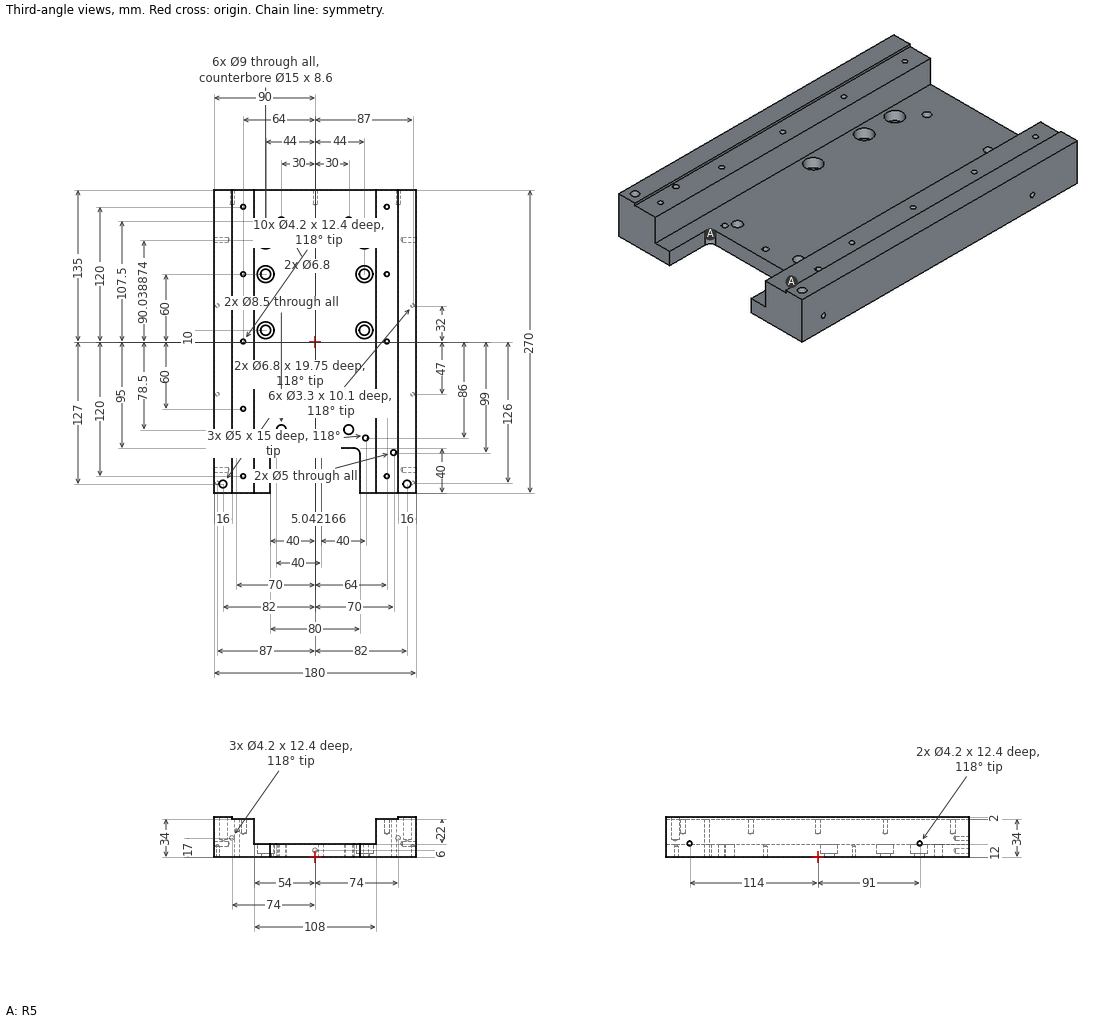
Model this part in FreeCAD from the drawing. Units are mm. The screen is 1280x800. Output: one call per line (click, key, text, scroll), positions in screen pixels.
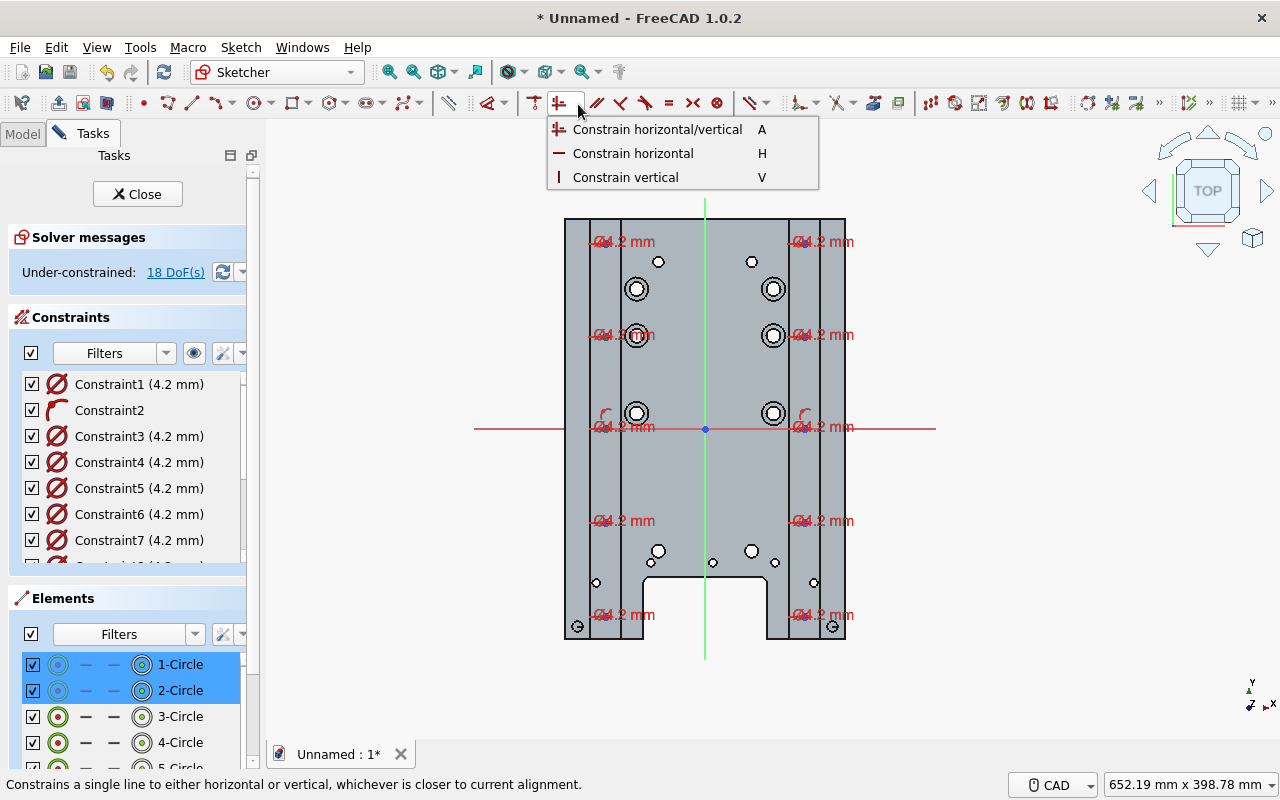
click(683, 177)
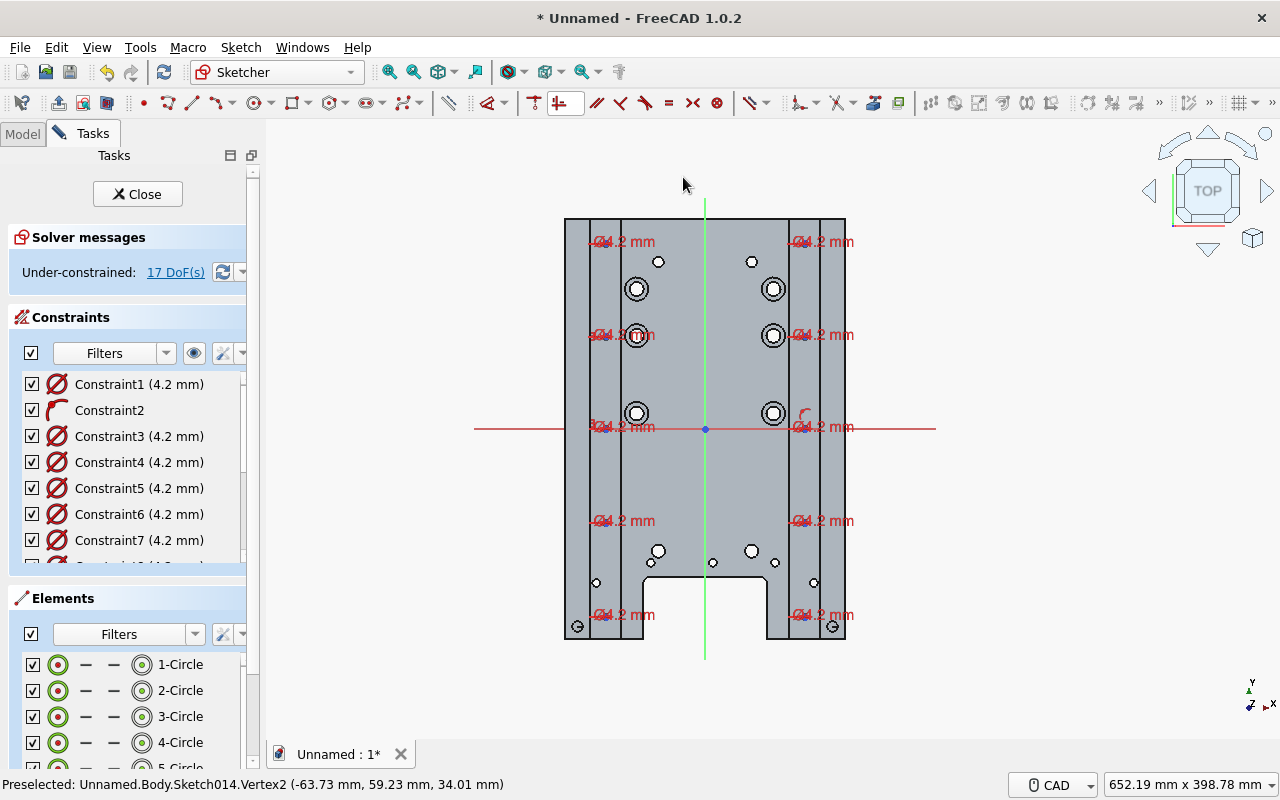
click(606, 337)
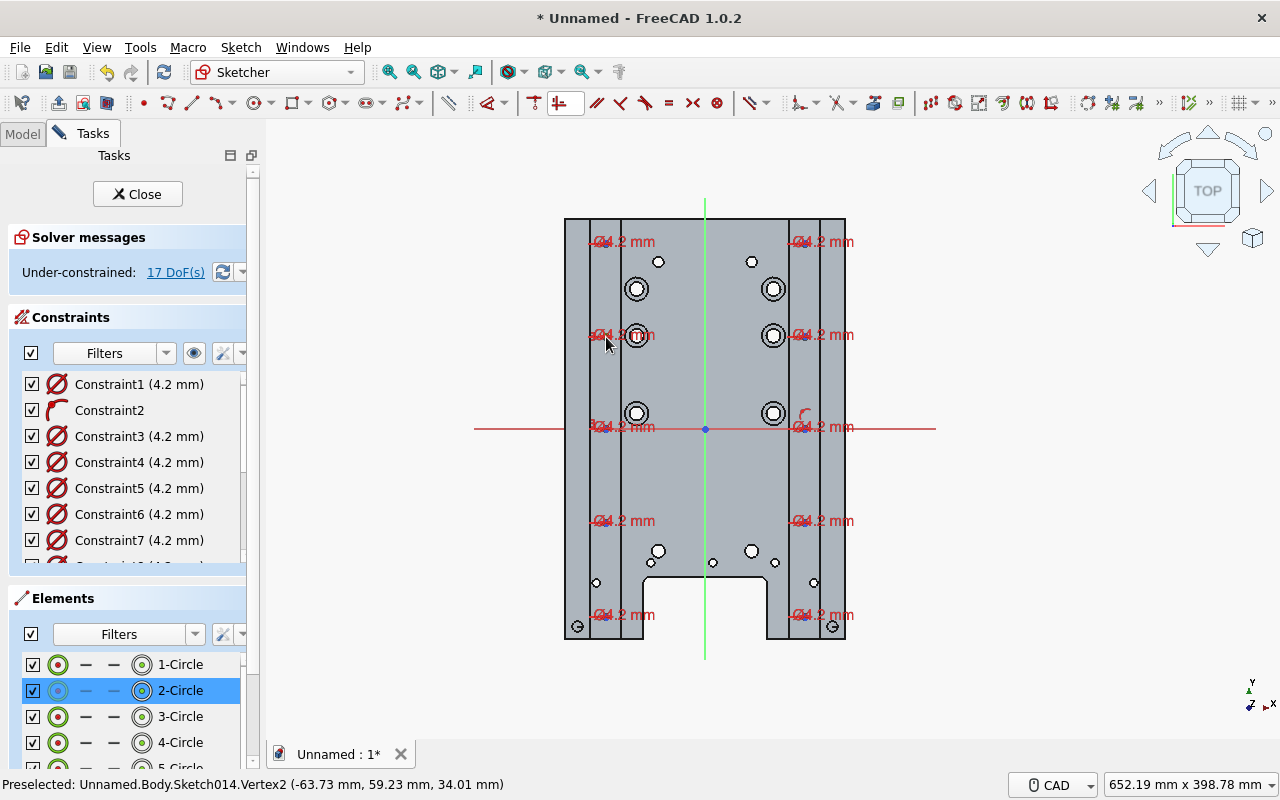
click(606, 244)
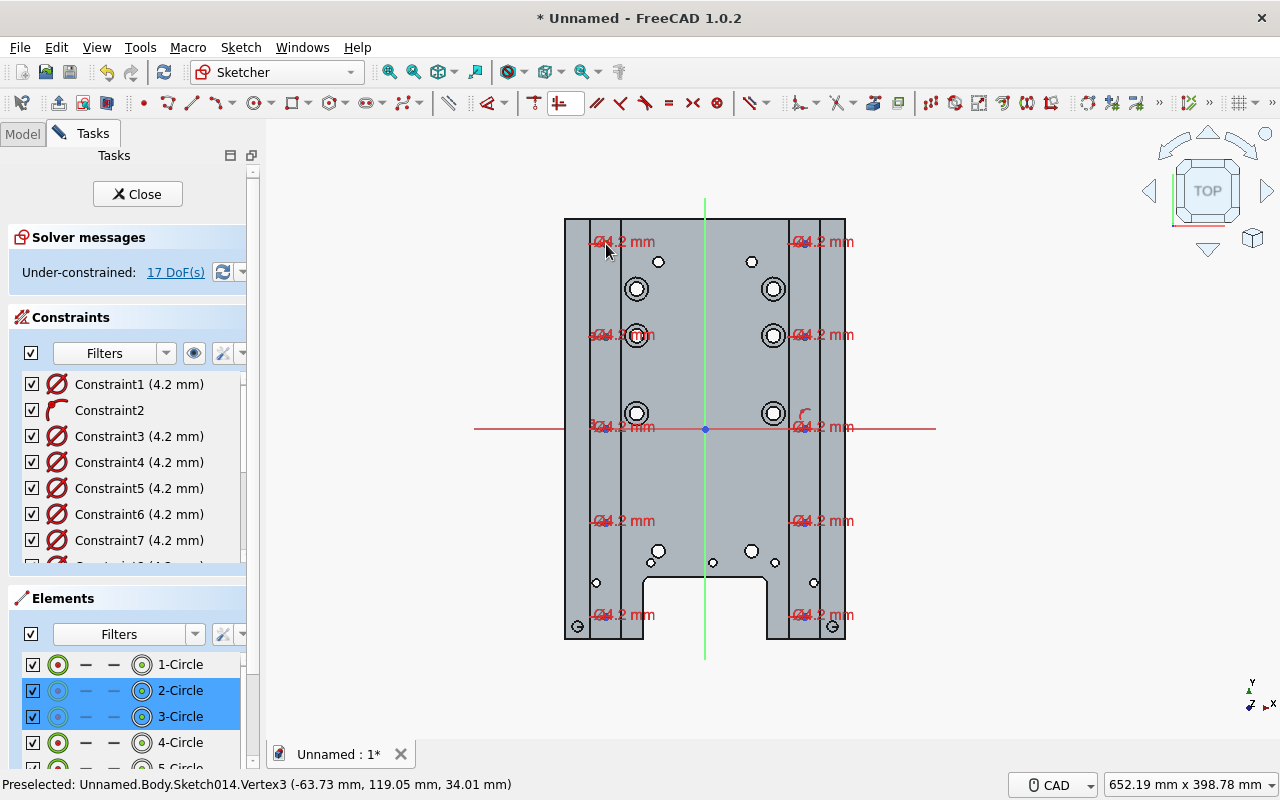
click(578, 104)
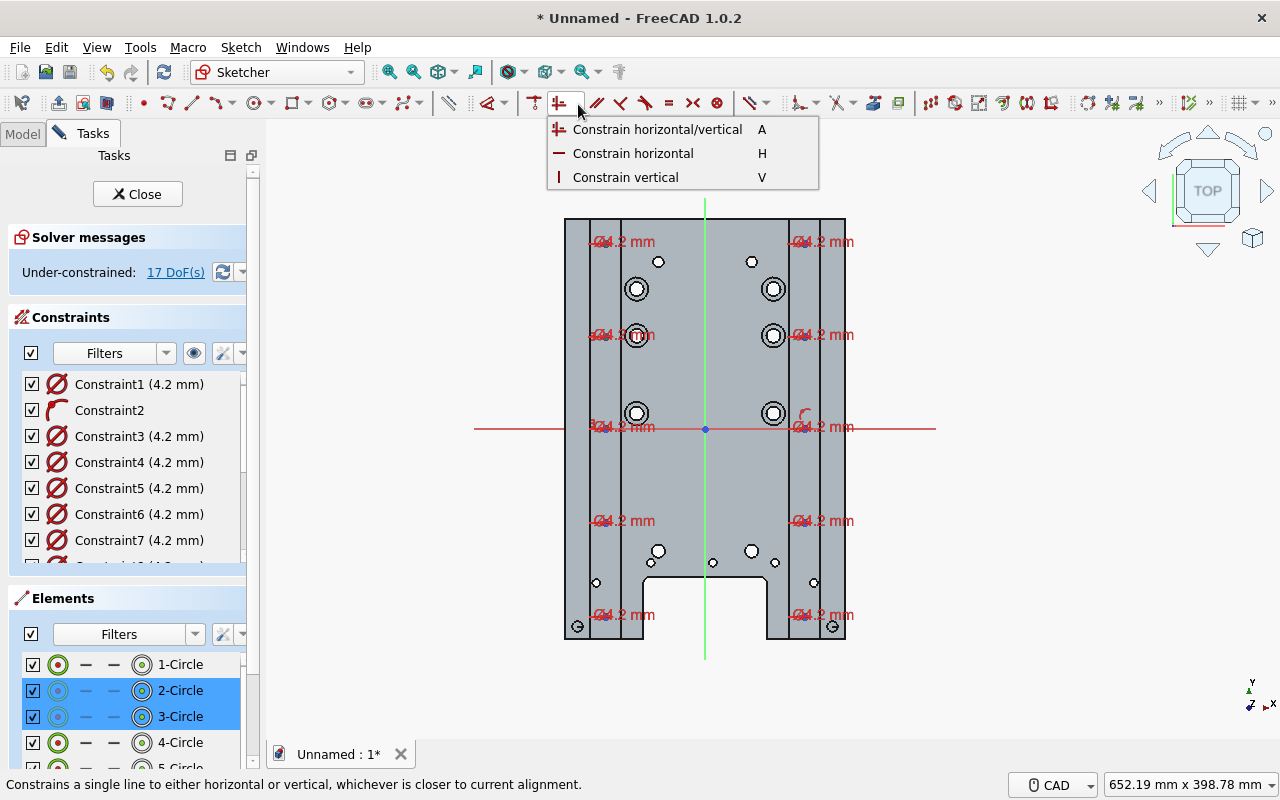
click(683, 177)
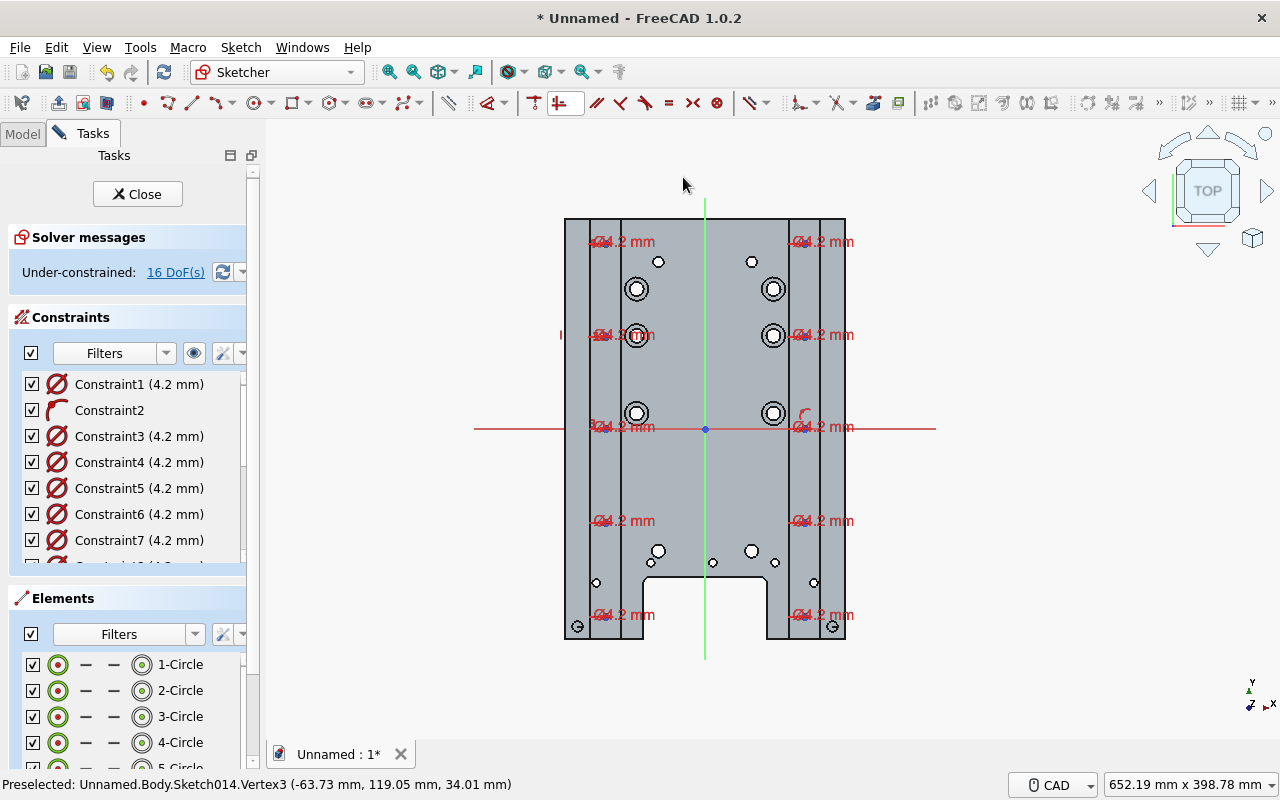
click(606, 429)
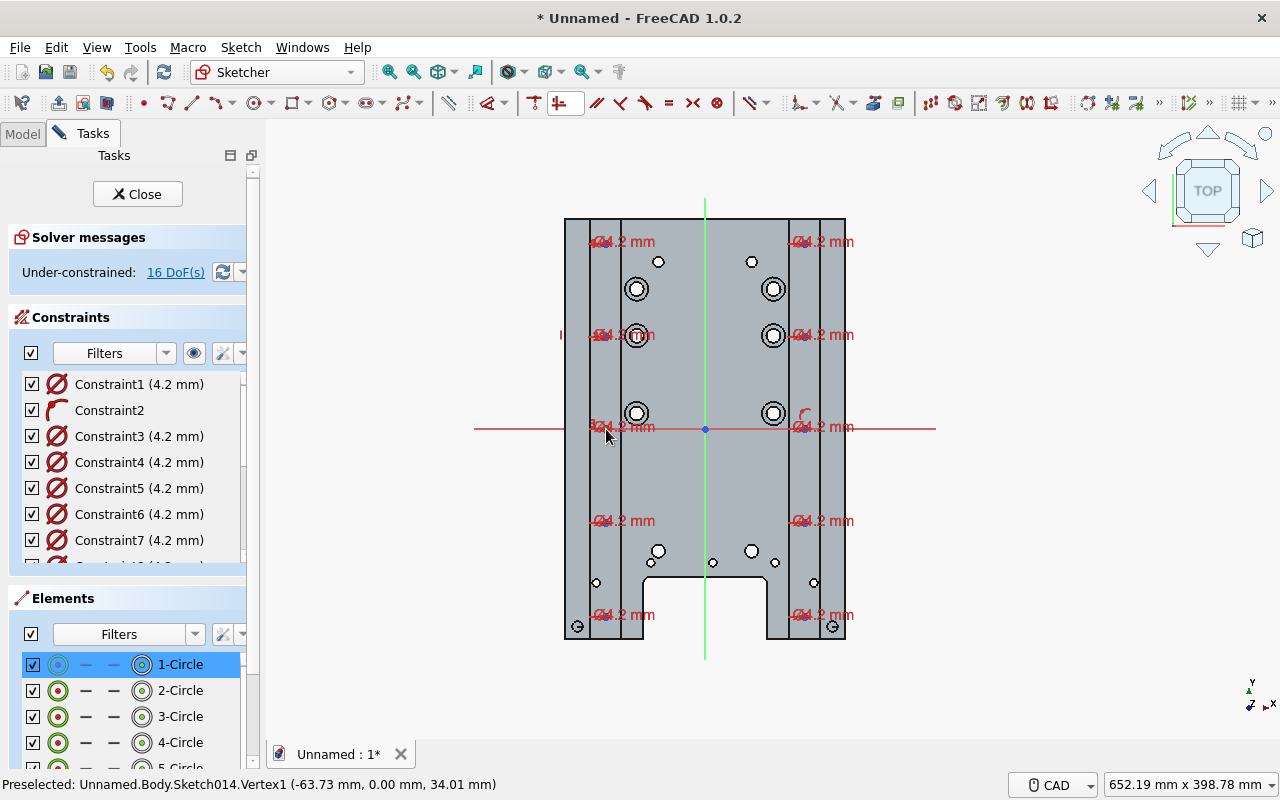
click(606, 617)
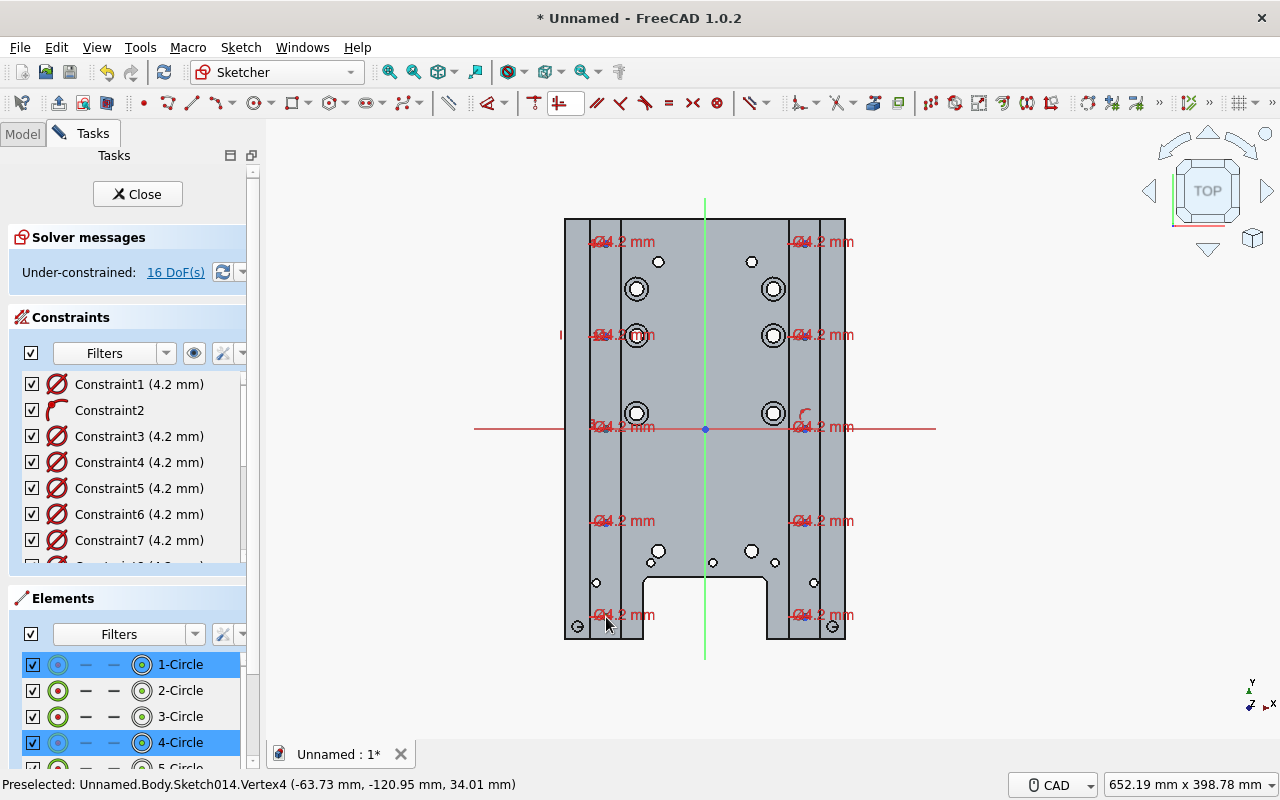
click(578, 104)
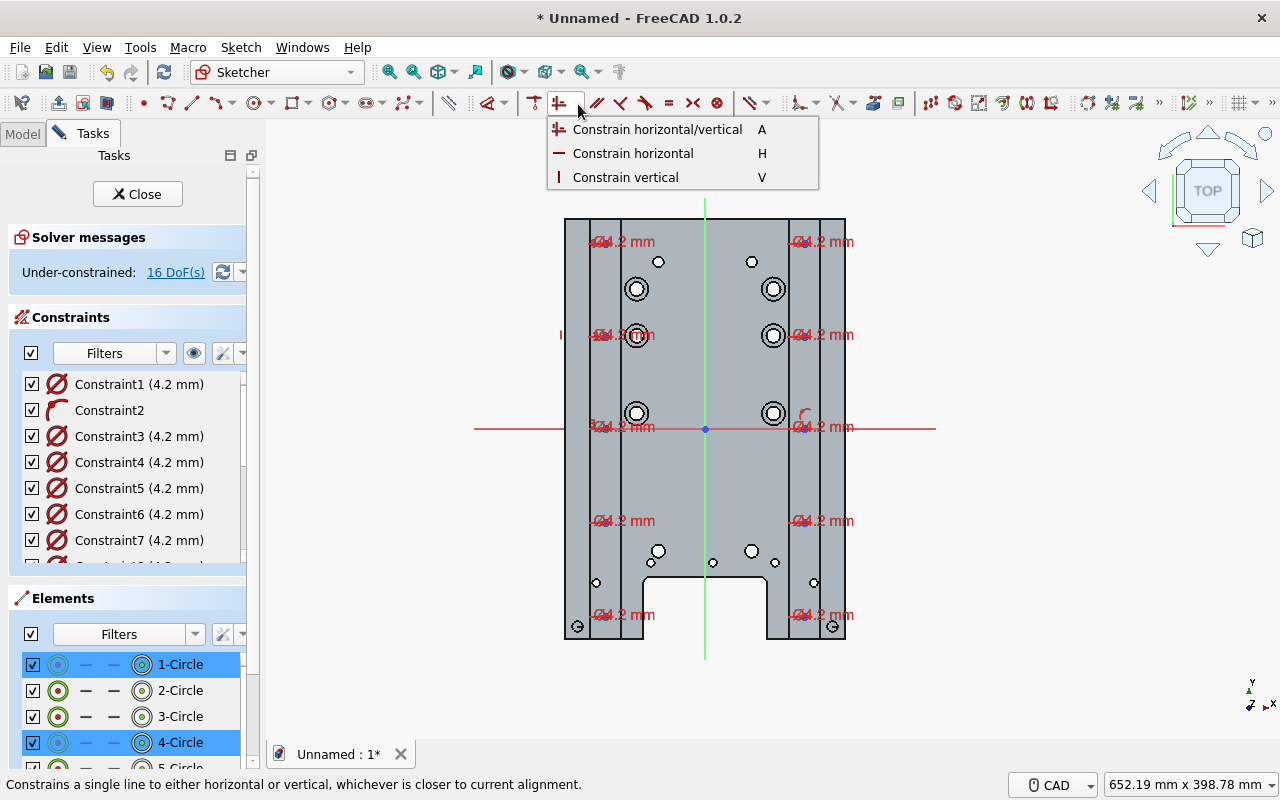
click(683, 177)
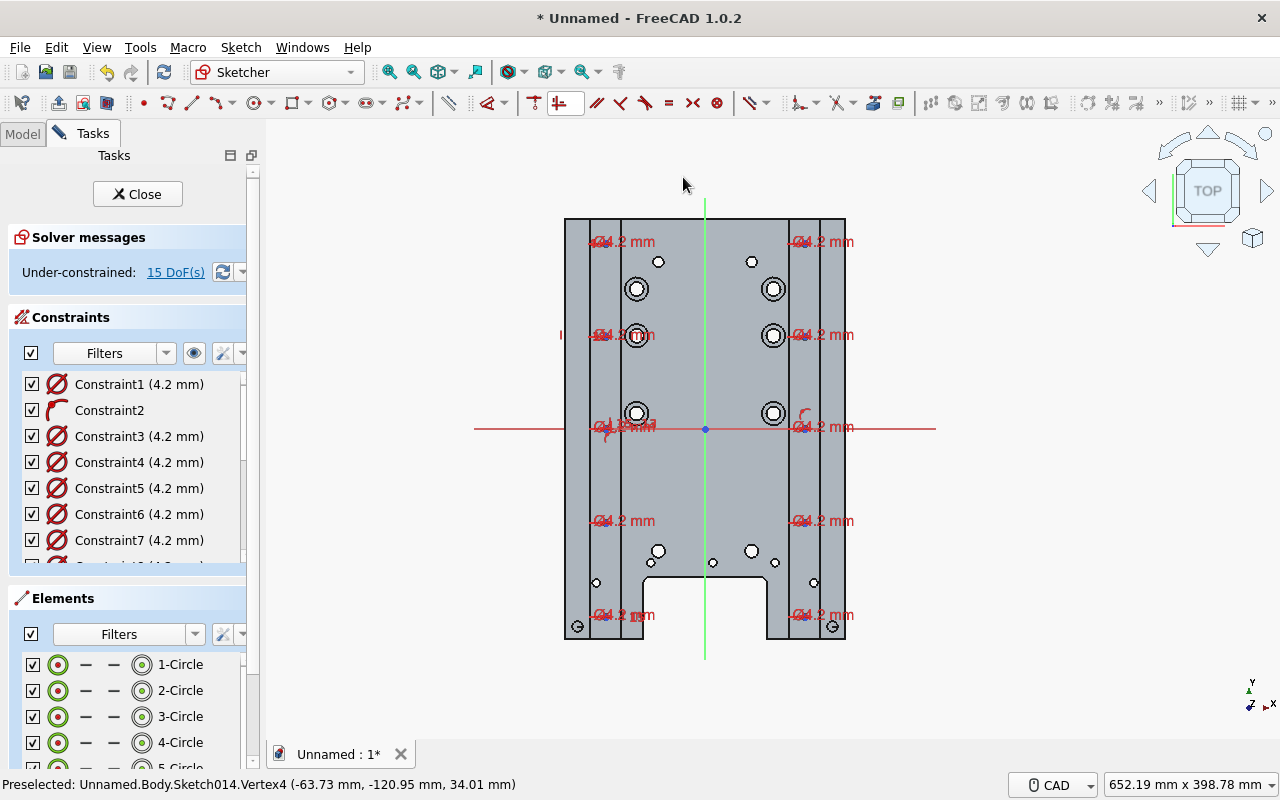
click(606, 429)